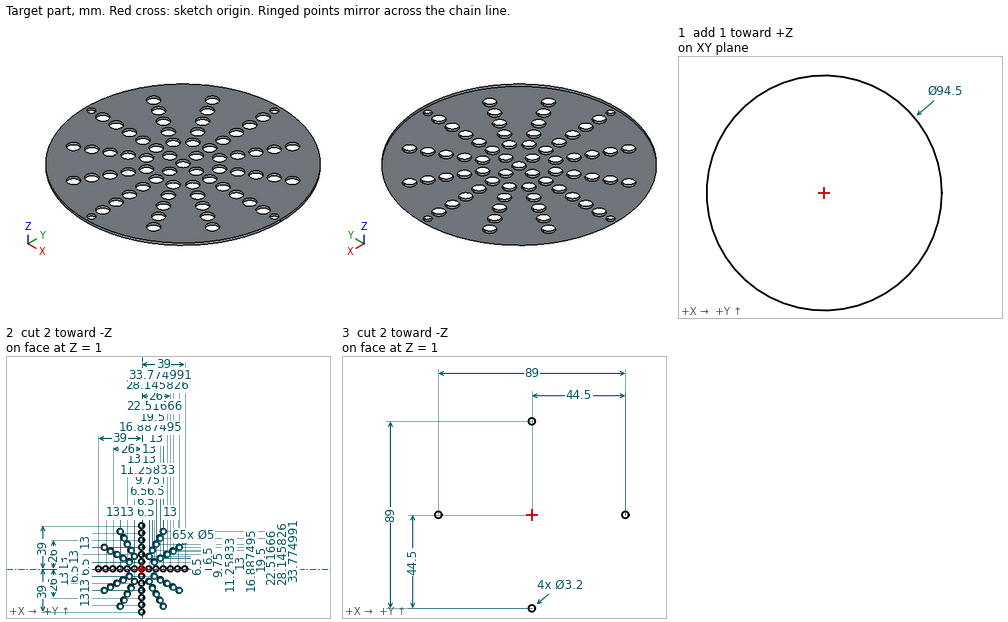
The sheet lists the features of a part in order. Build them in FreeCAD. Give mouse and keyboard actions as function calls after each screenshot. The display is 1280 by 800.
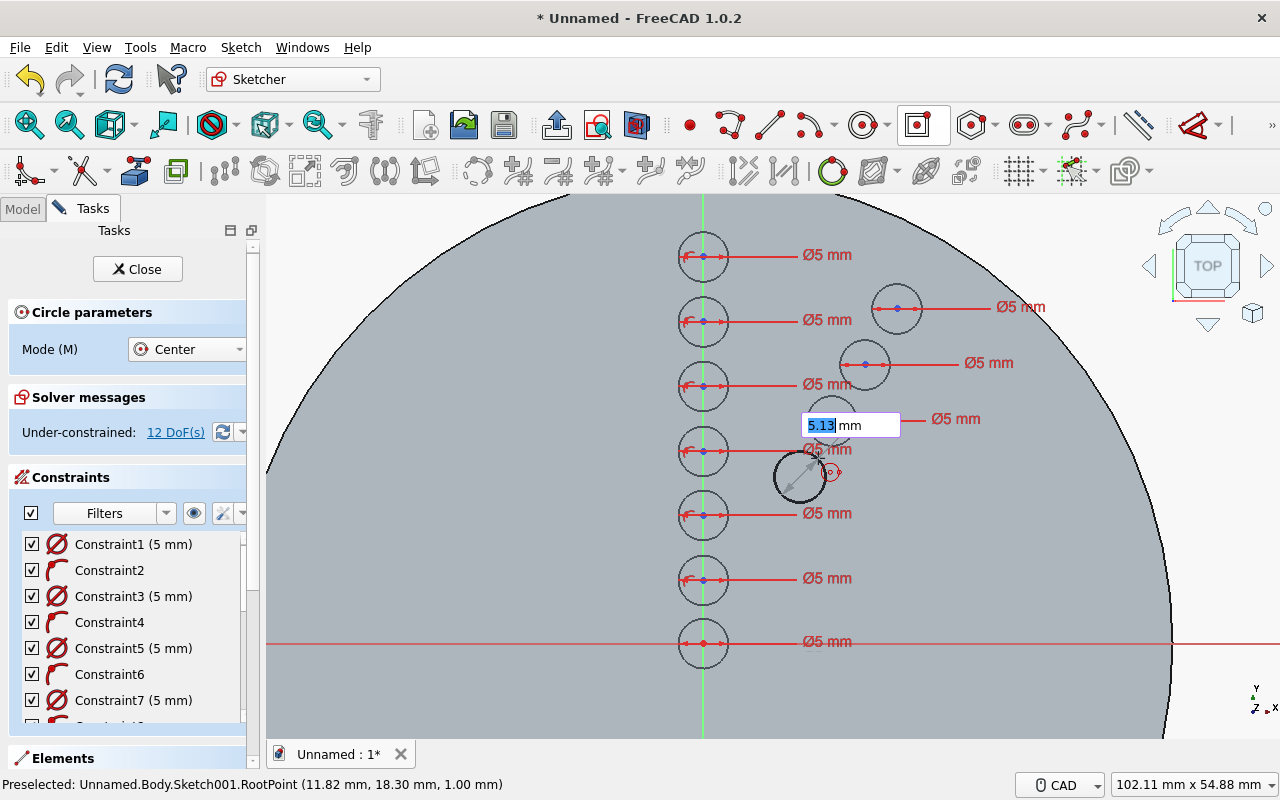
text(5)
key(Return)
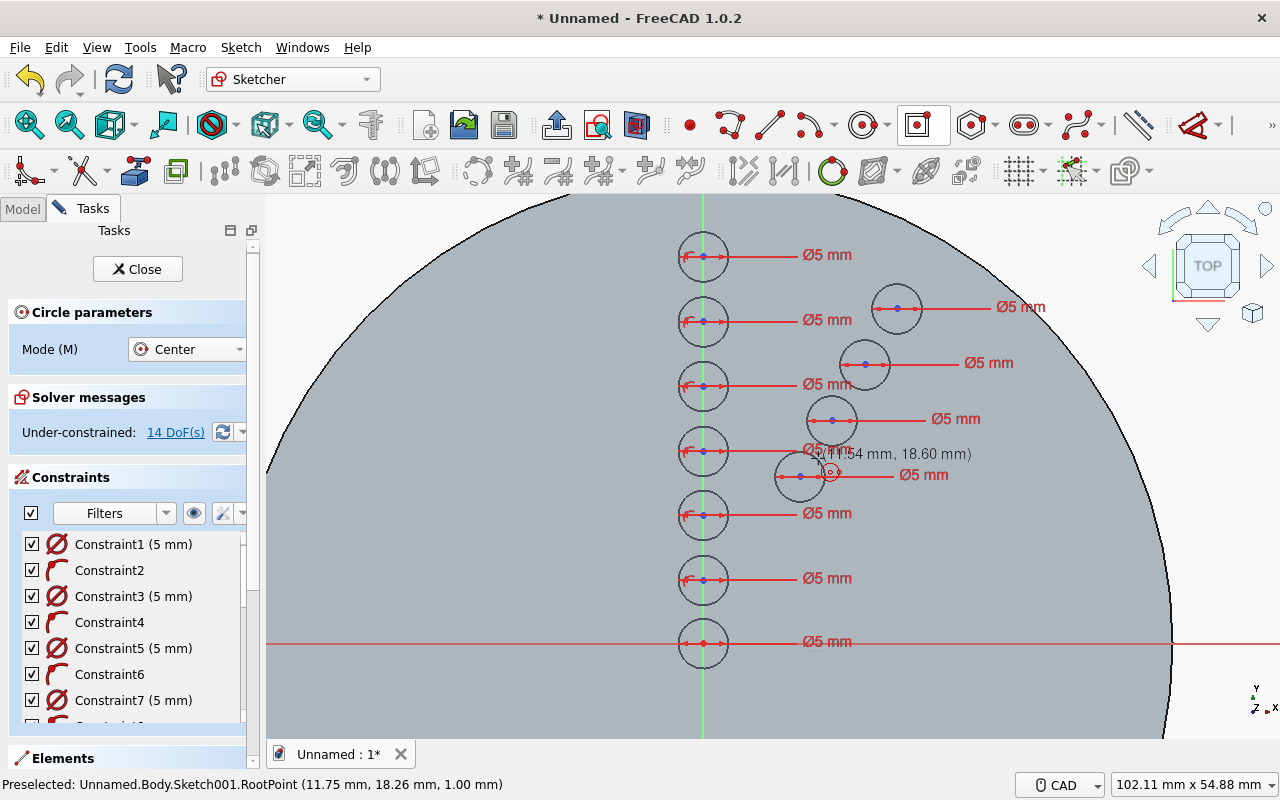
click(768, 532)
move(785, 514)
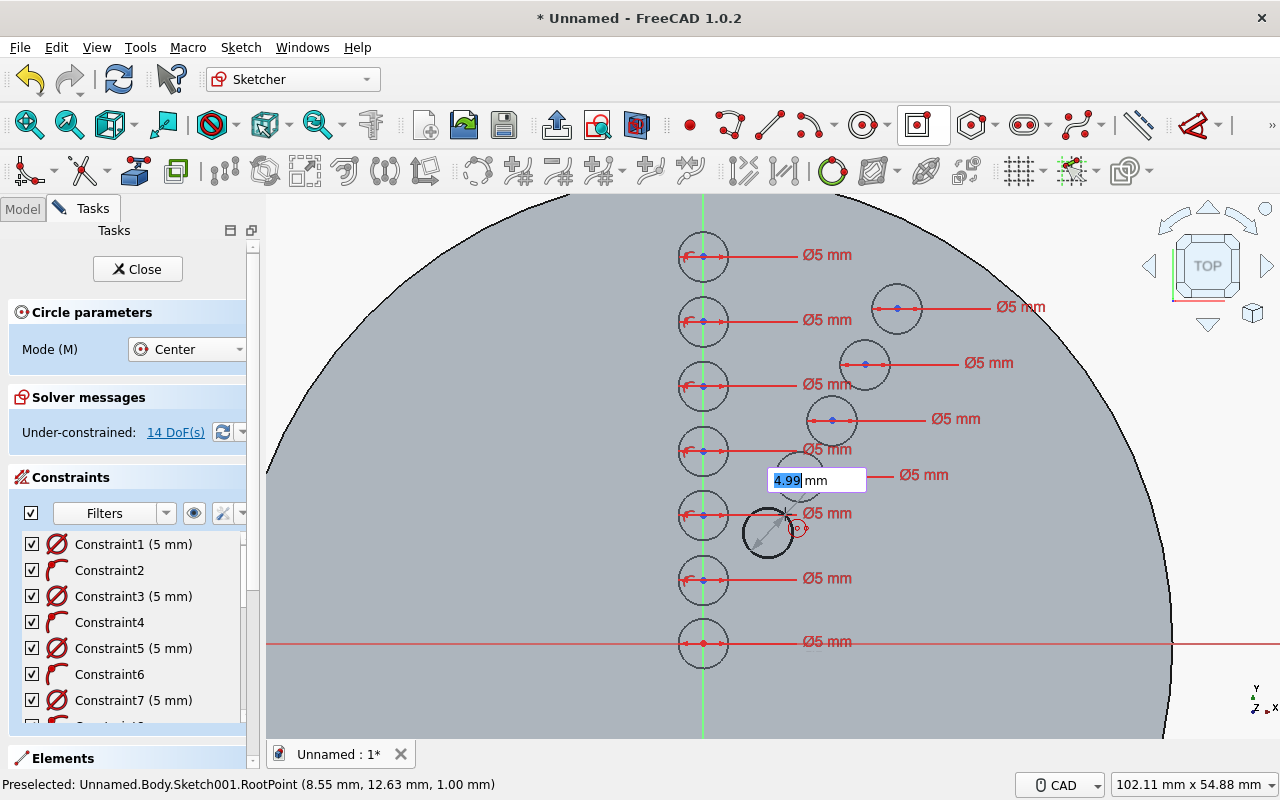
text(5)
key(Return)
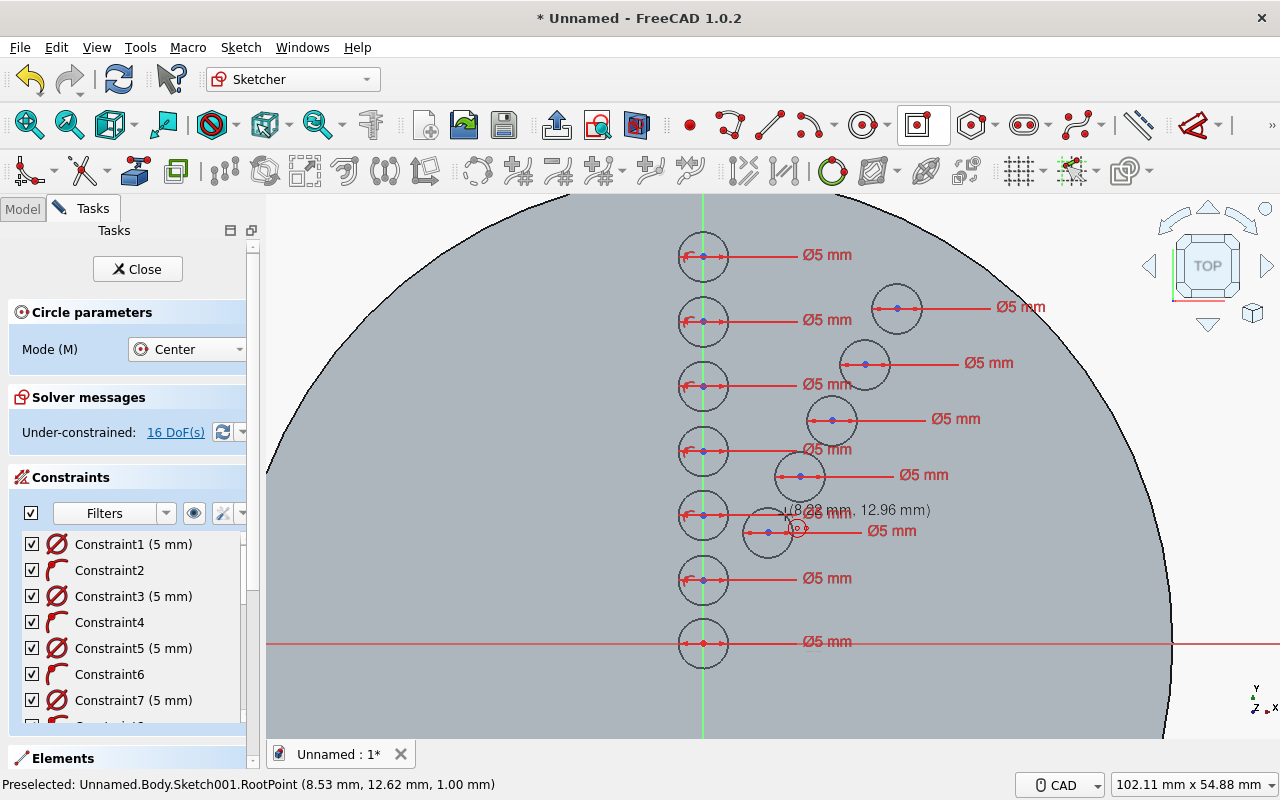
click(1039, 450)
move(1056, 433)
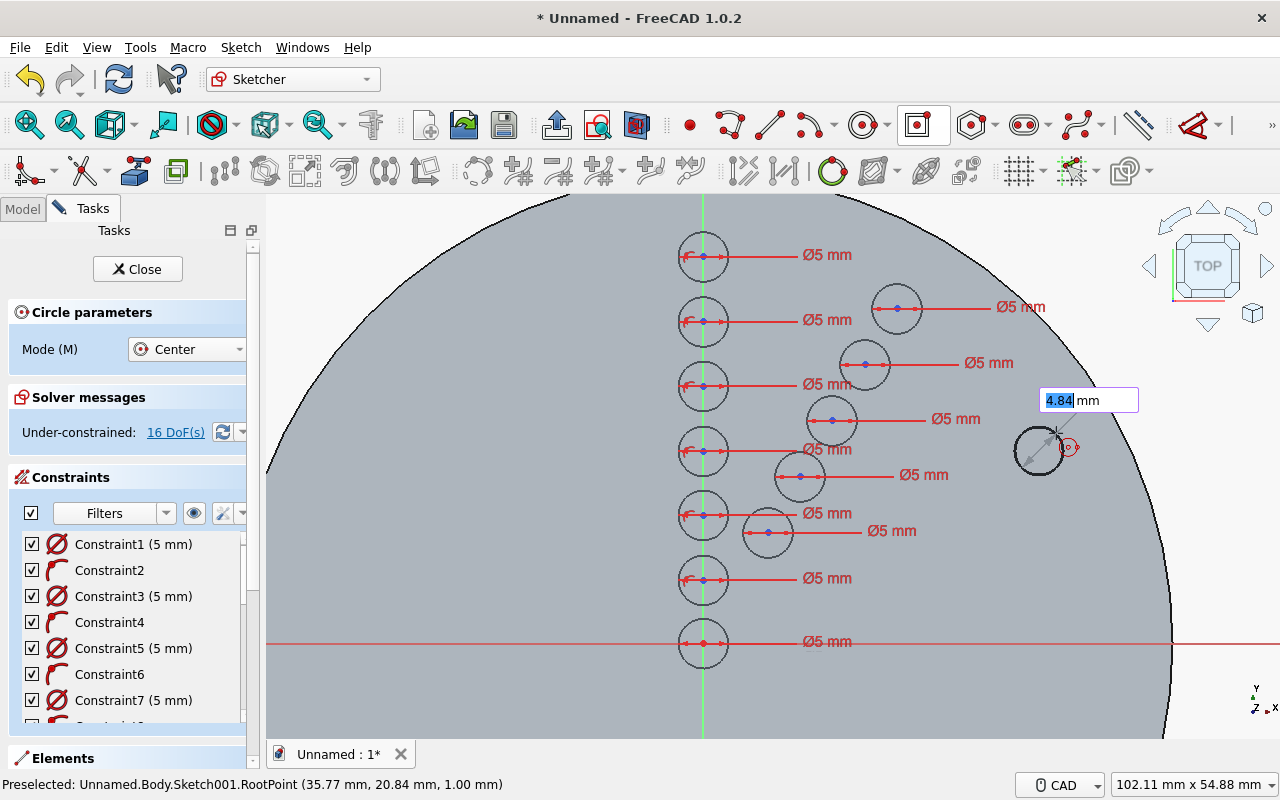
text(5)
key(Return)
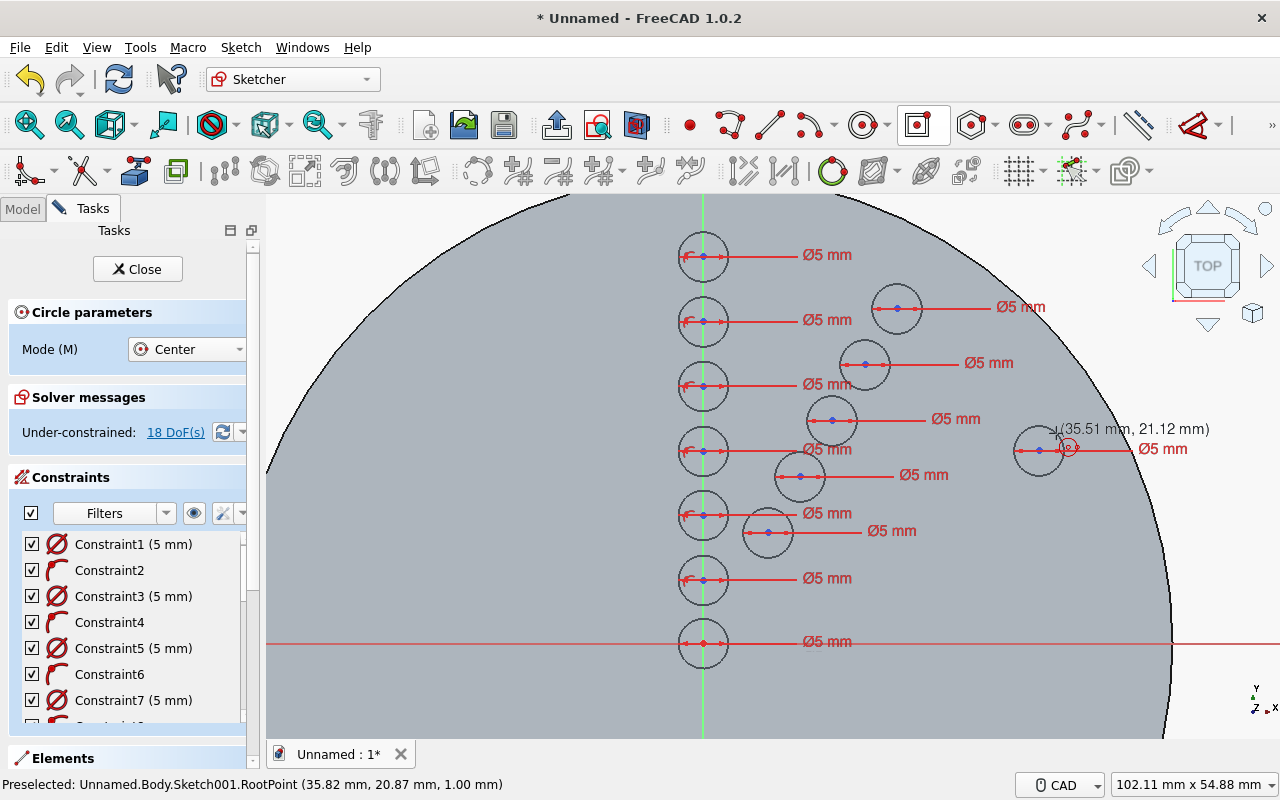
click(983, 482)
move(1000, 465)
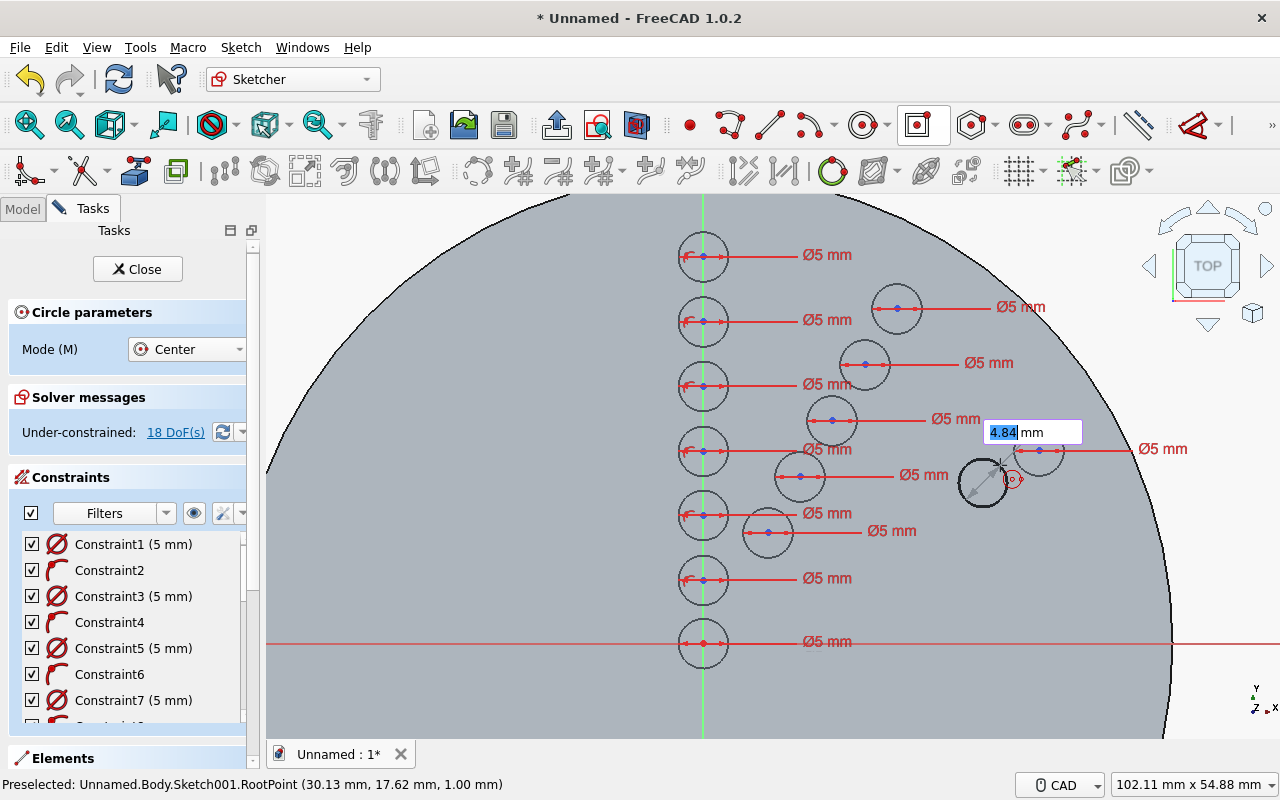
text(5)
key(Return)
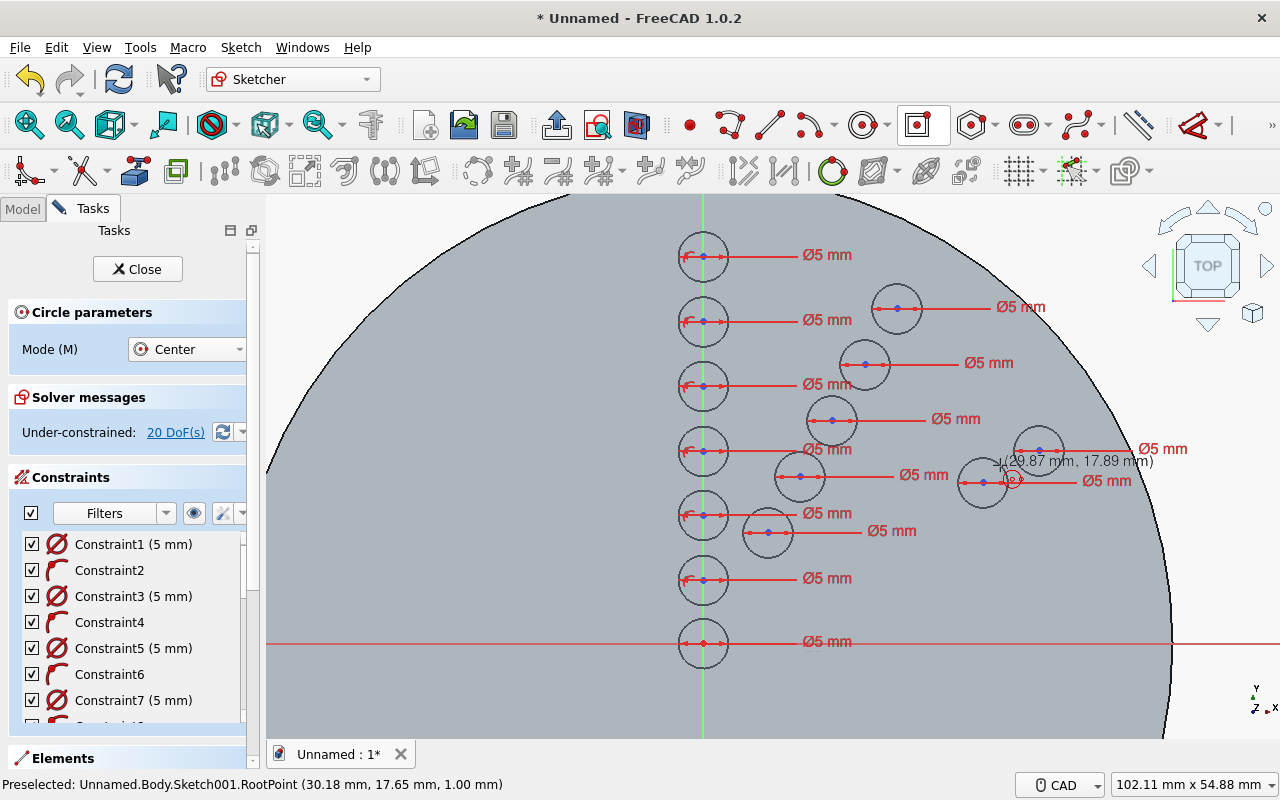
click(927, 515)
move(945, 497)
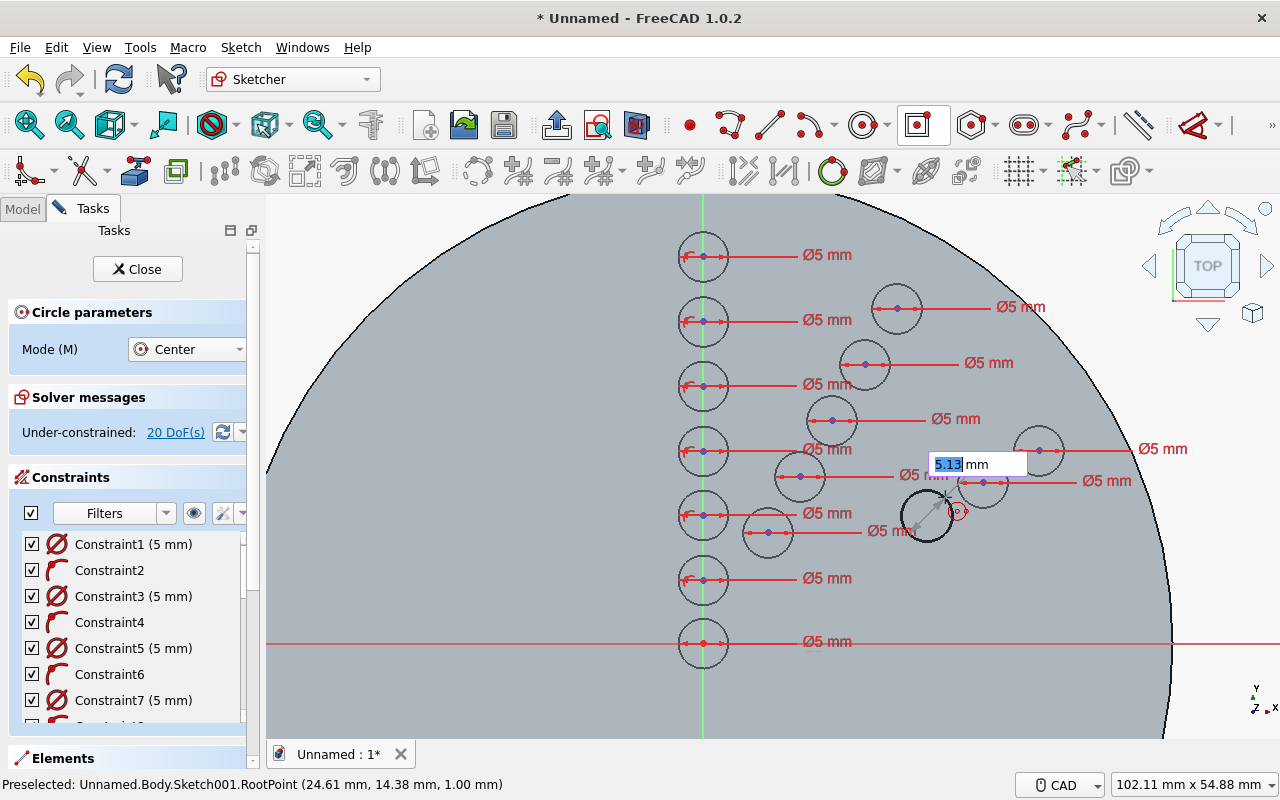
text(5)
key(Return)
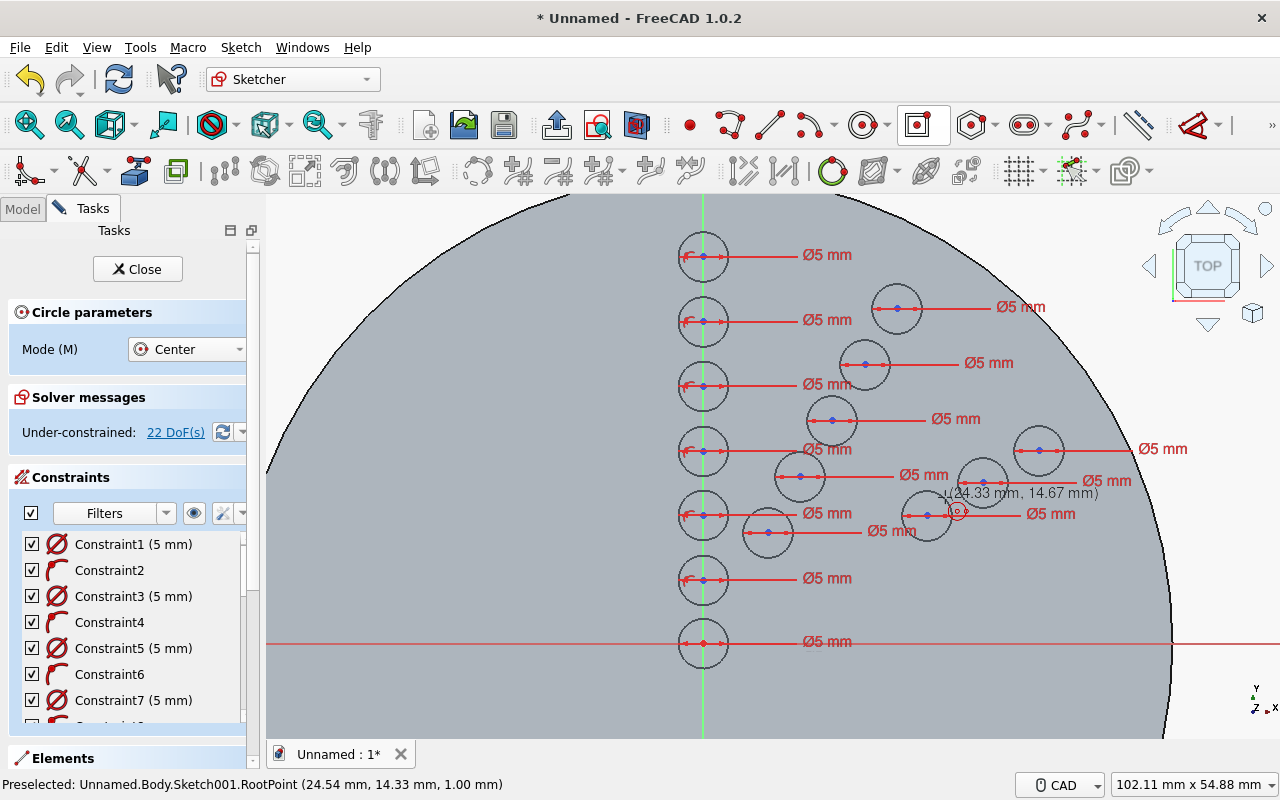
click(871, 547)
move(889, 529)